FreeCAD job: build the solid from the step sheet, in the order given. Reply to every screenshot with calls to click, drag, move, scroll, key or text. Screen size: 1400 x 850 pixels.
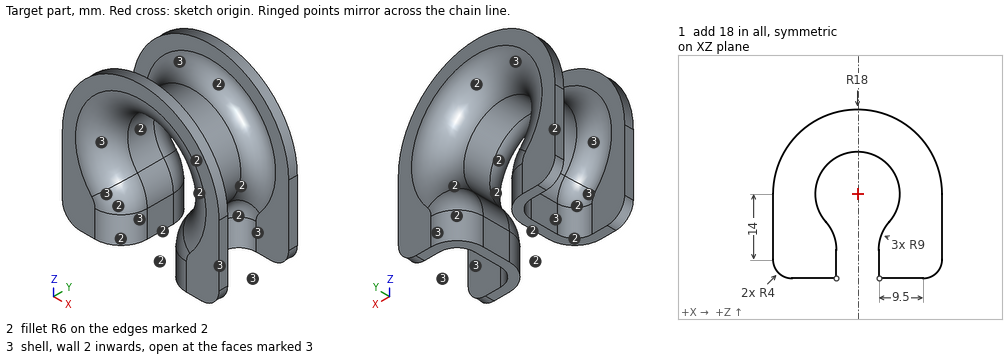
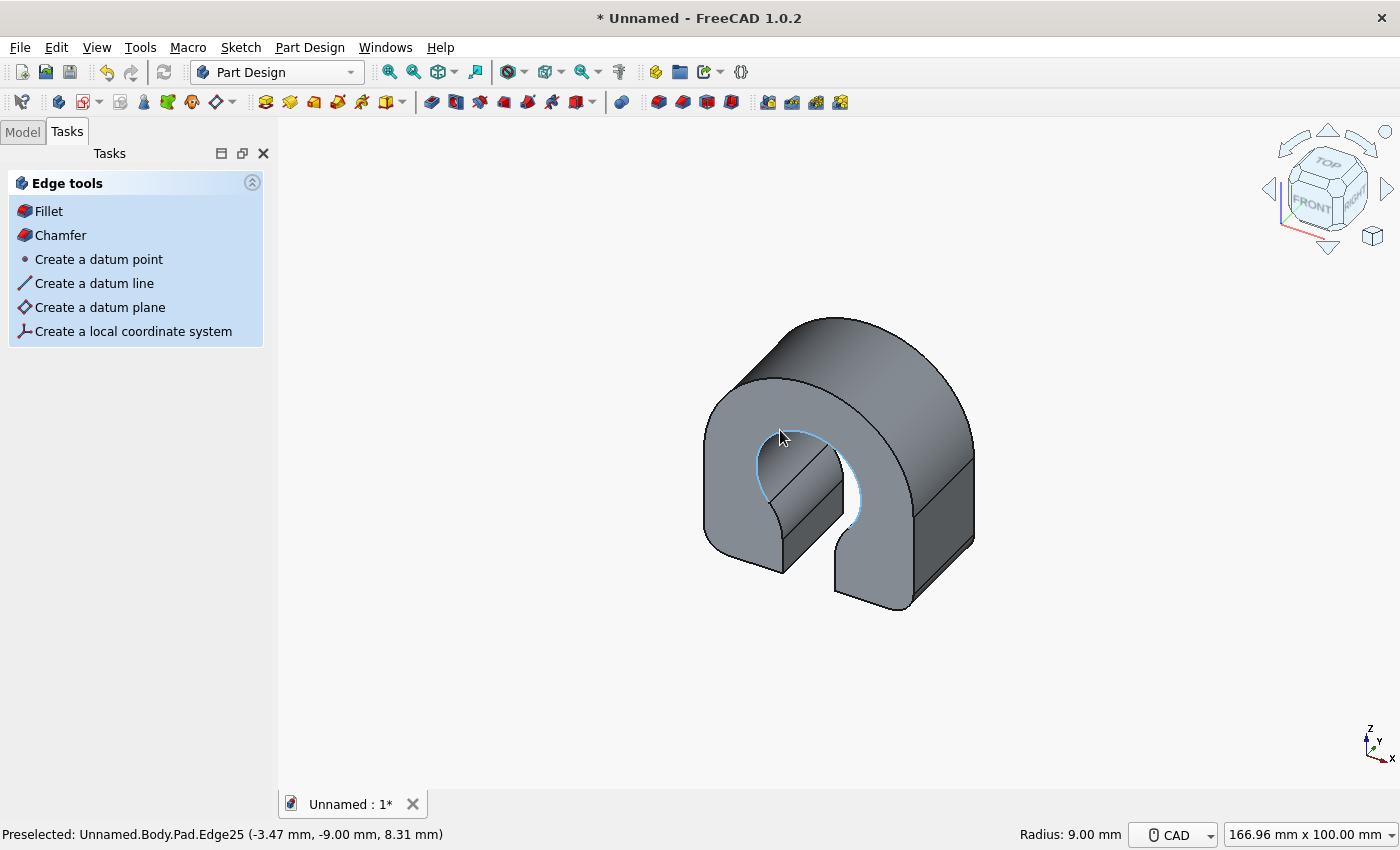
click(842, 534, ctrl)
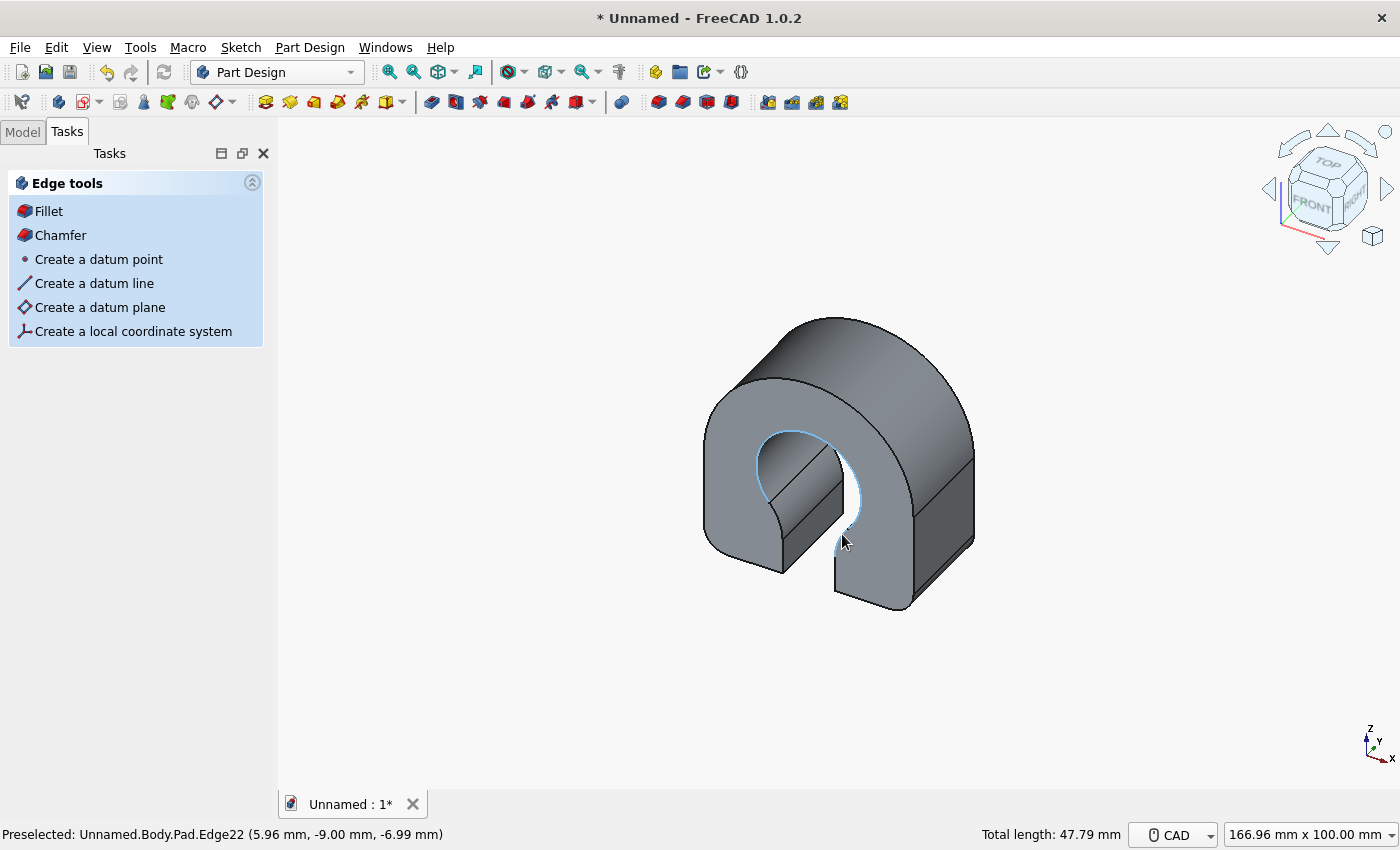
click(783, 556, ctrl)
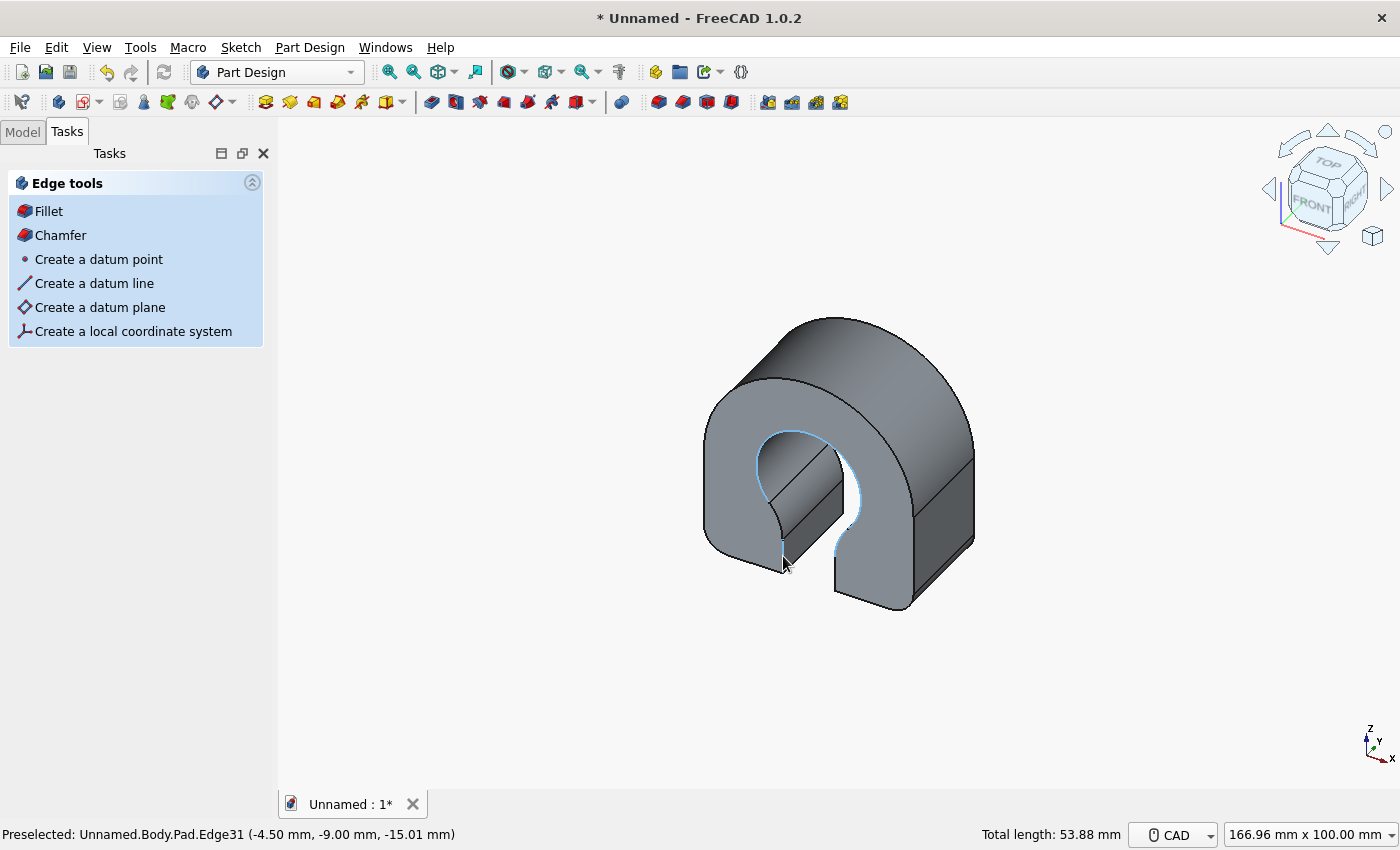
click(779, 520, ctrl)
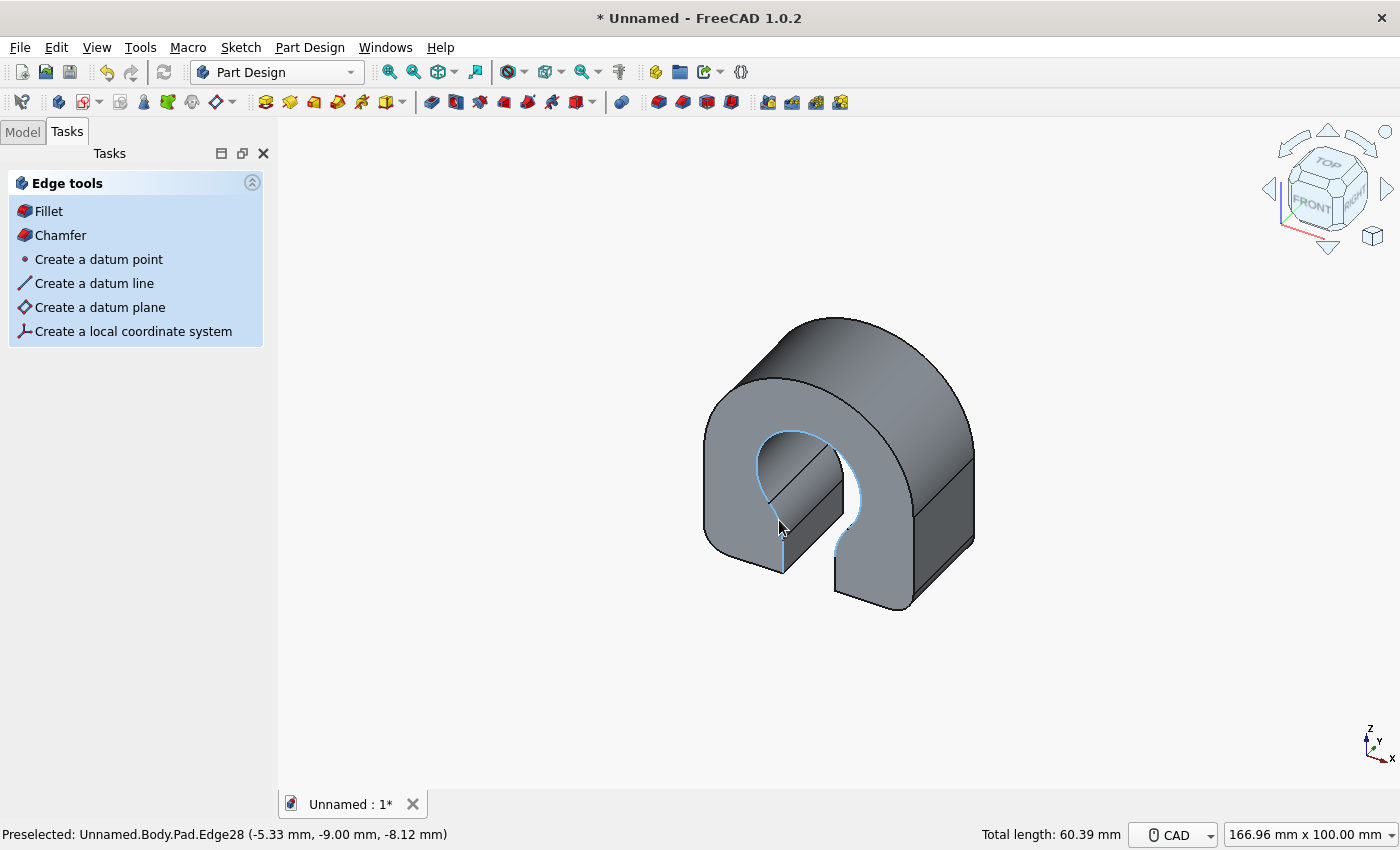
key(0)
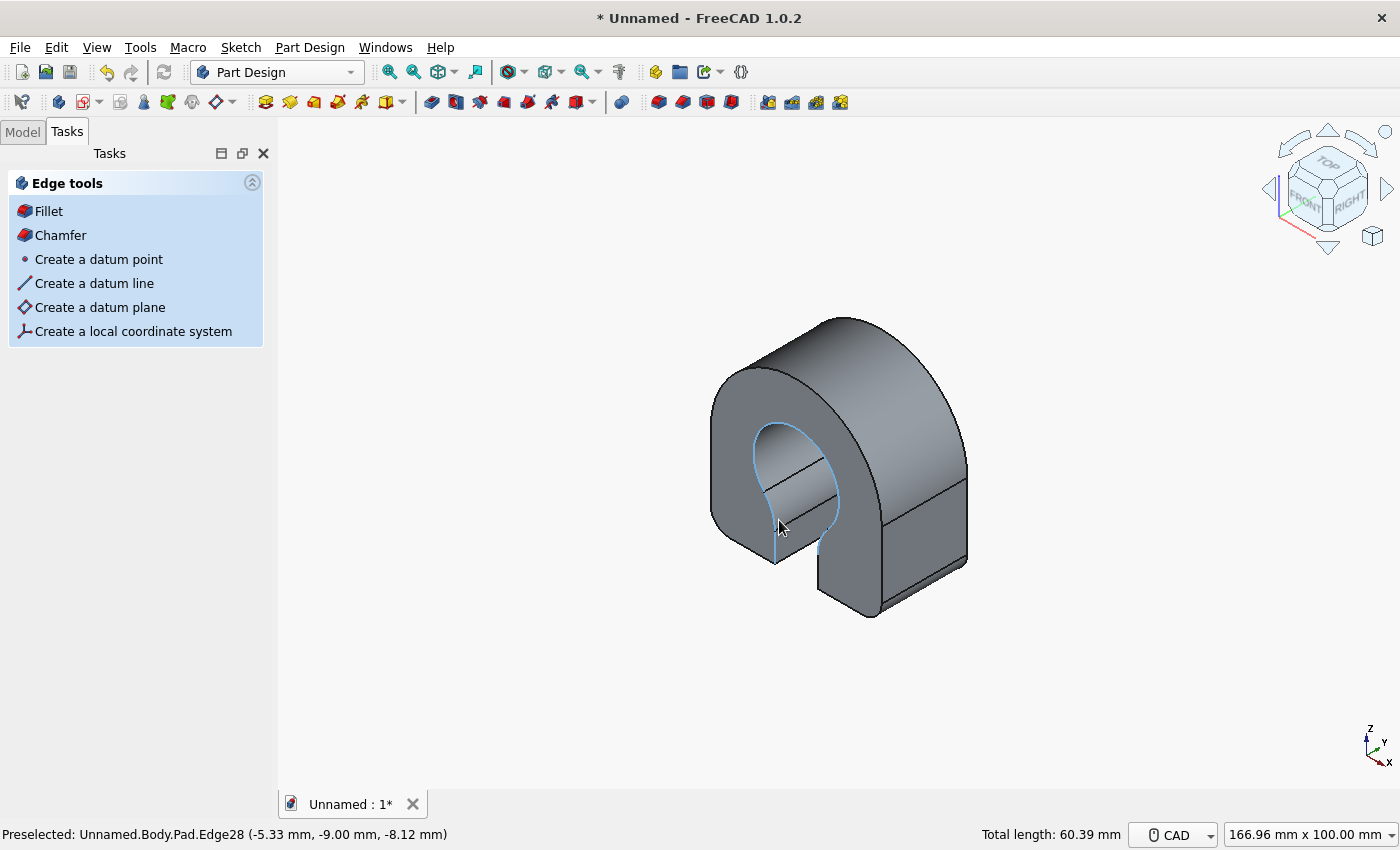
key(2)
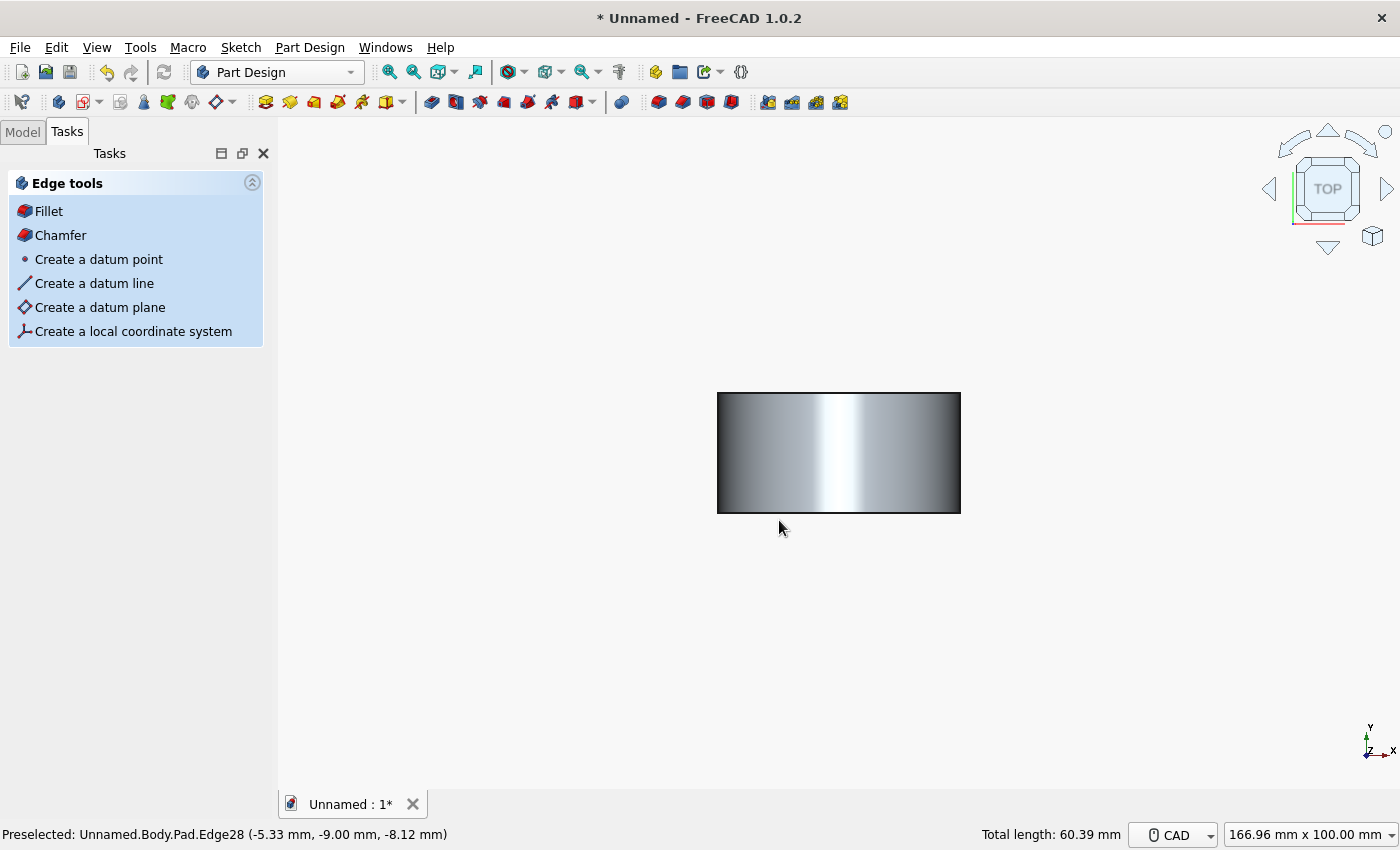
key(v)
key(f)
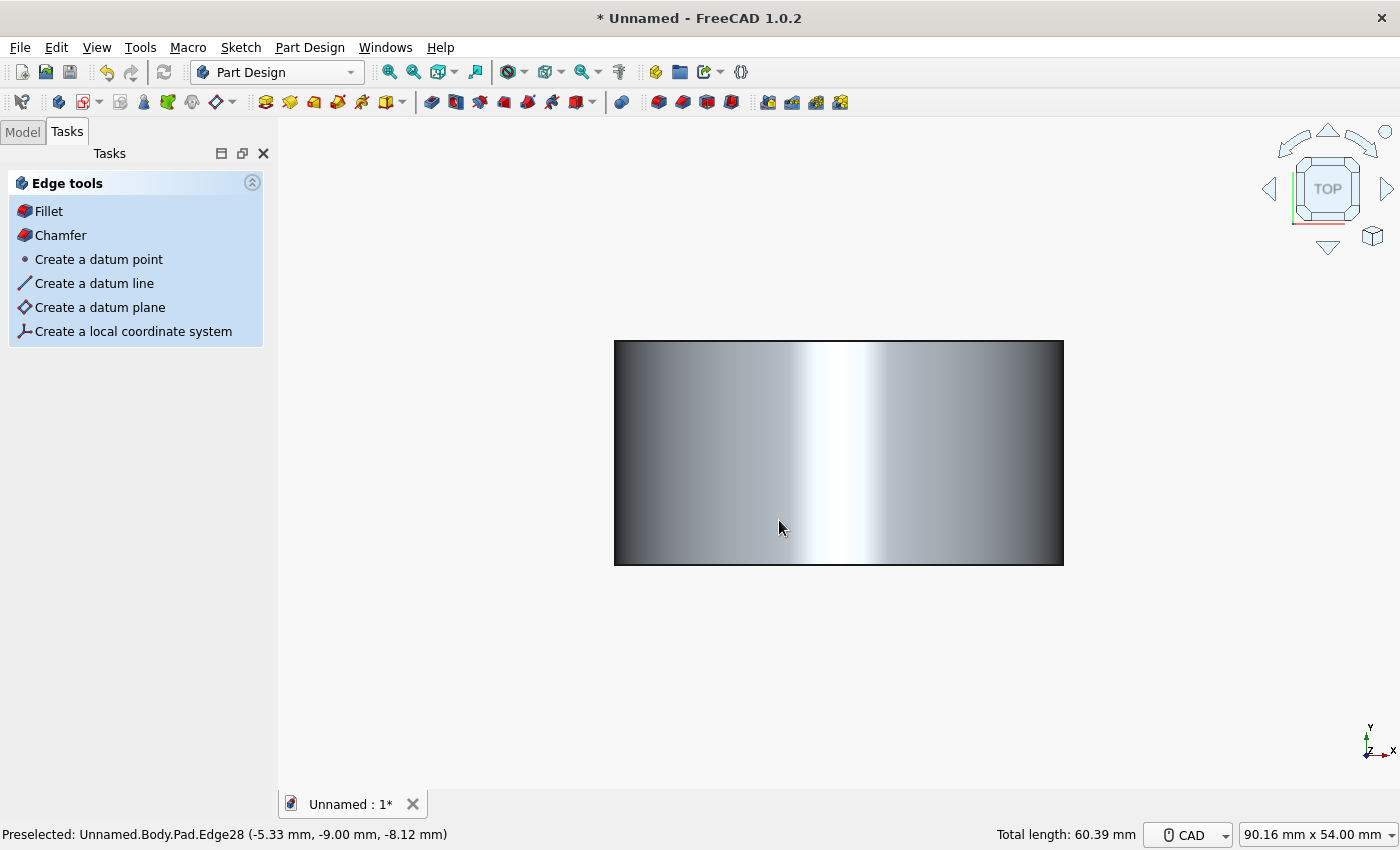
key(1)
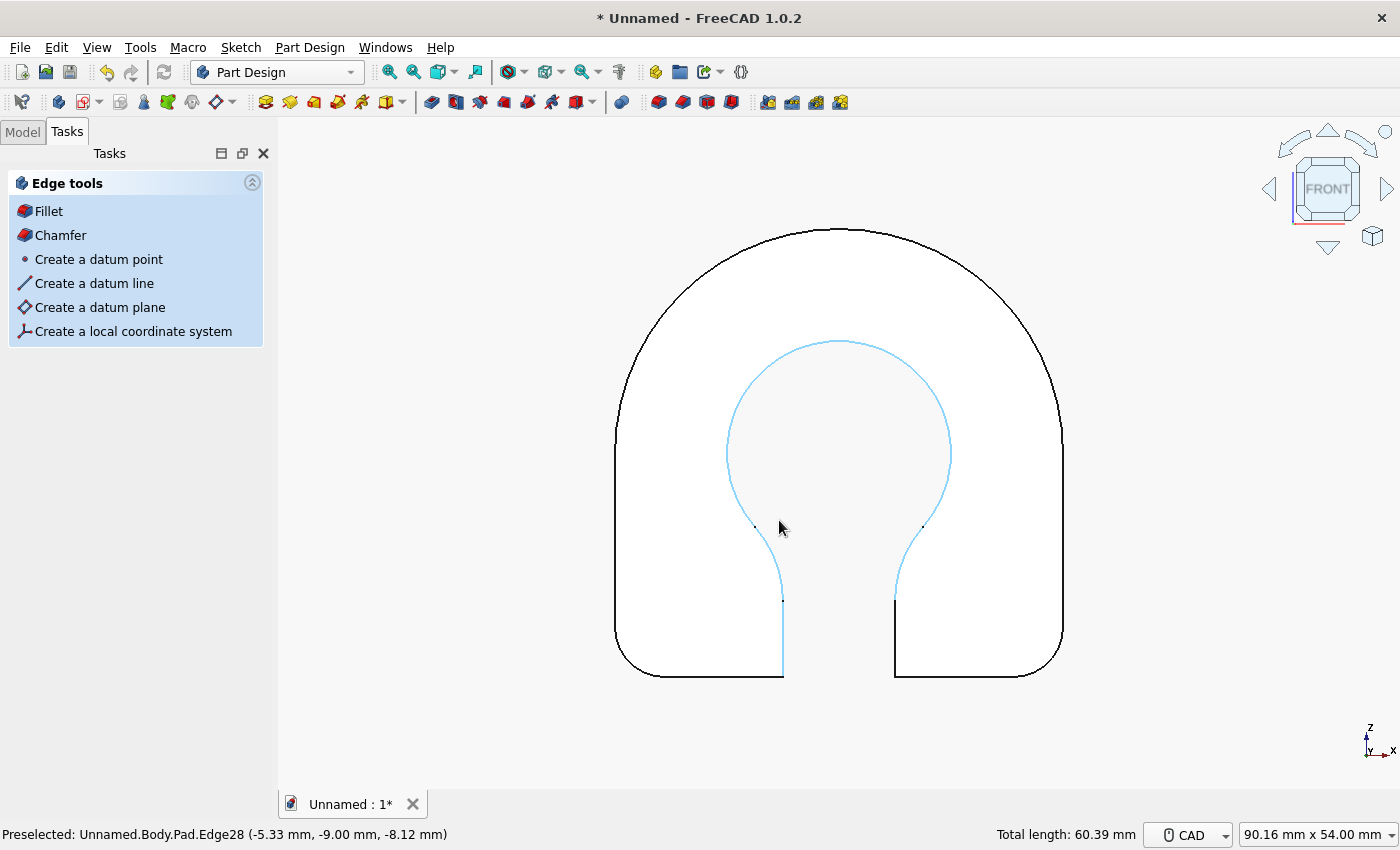
click(895, 638, ctrl)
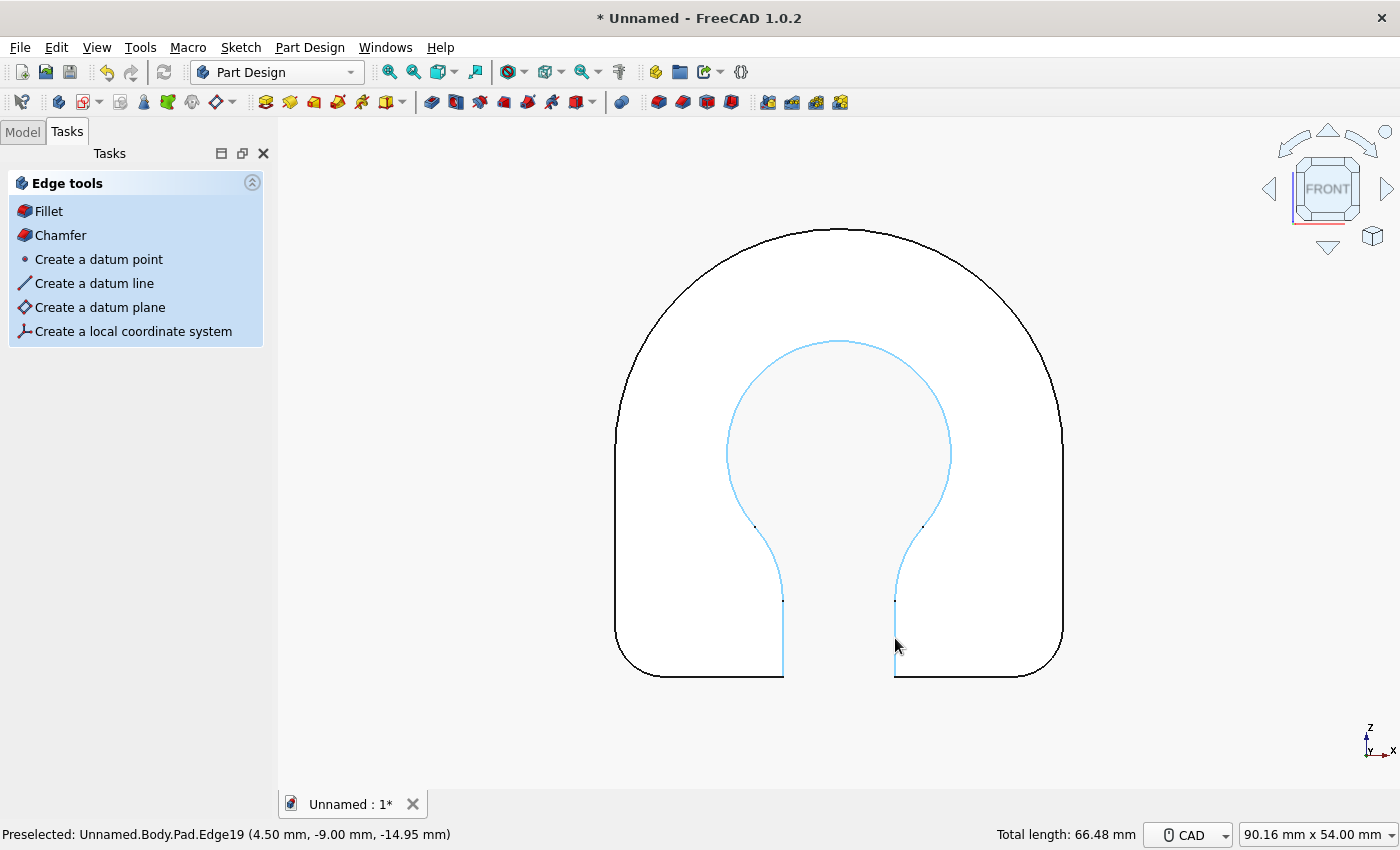
key(3)